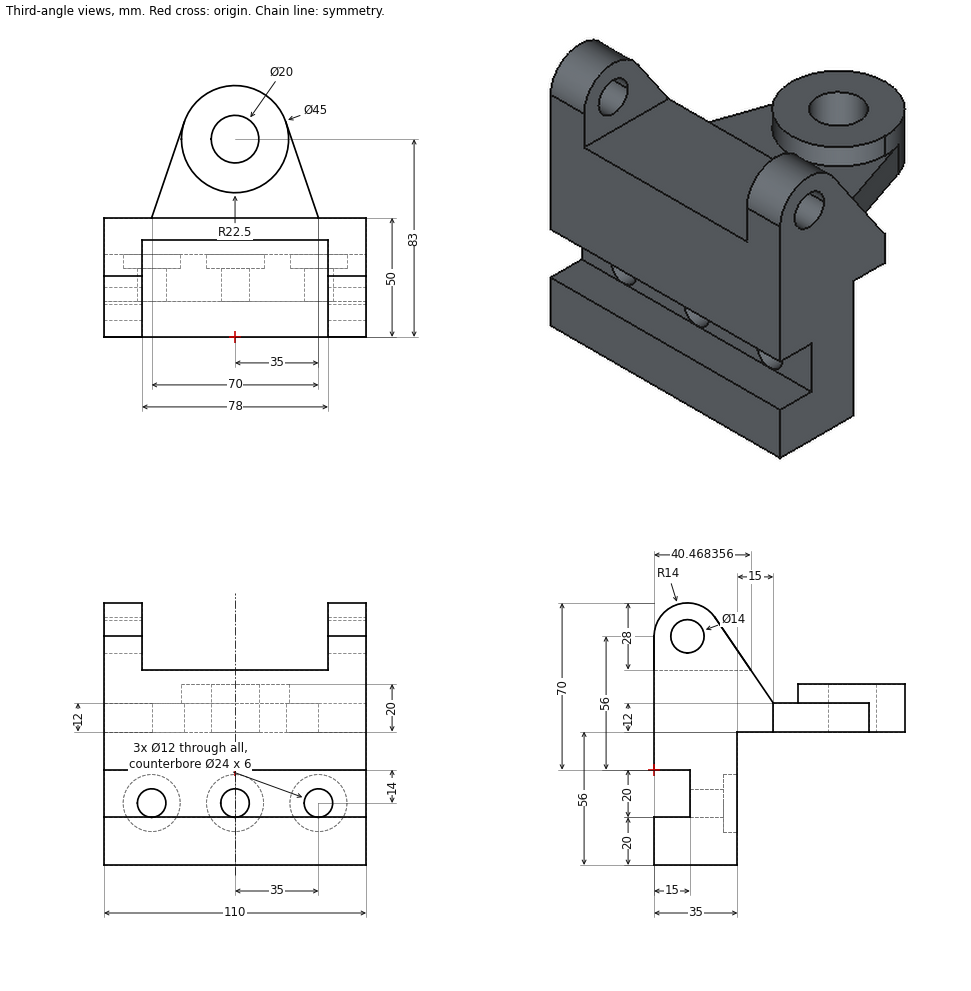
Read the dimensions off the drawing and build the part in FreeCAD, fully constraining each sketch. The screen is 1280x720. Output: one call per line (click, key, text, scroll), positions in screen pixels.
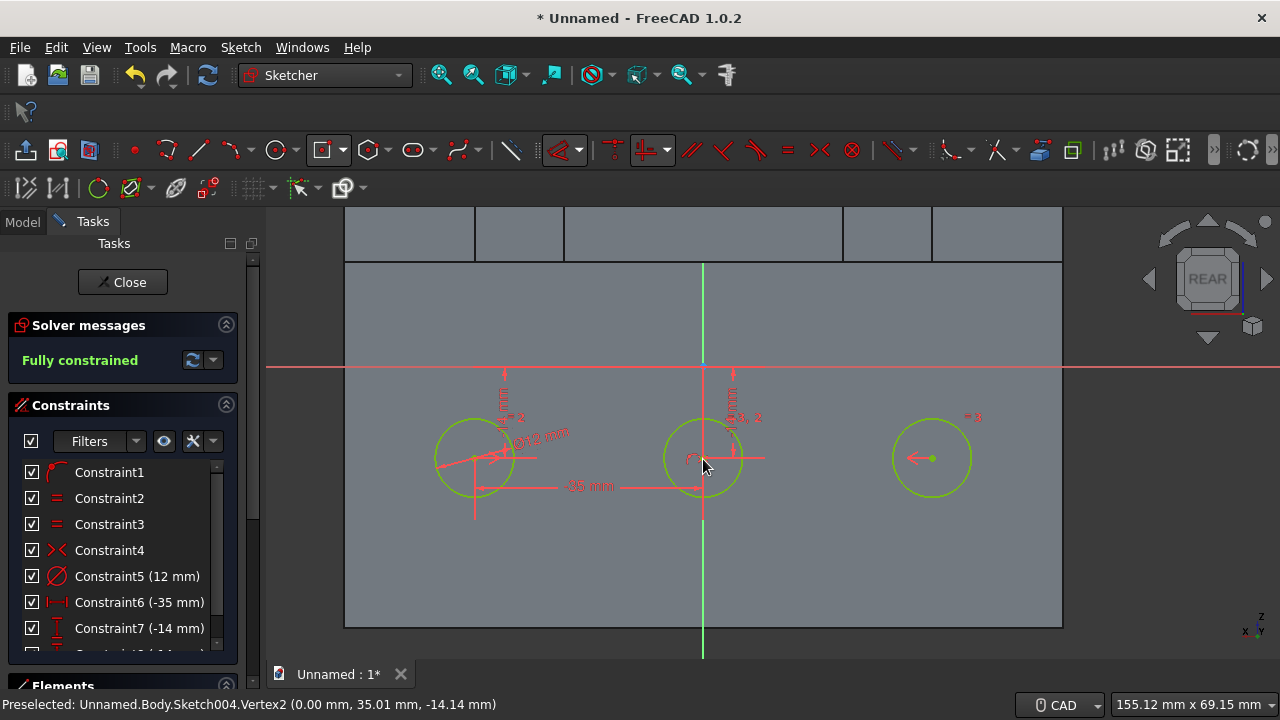
click(123, 282)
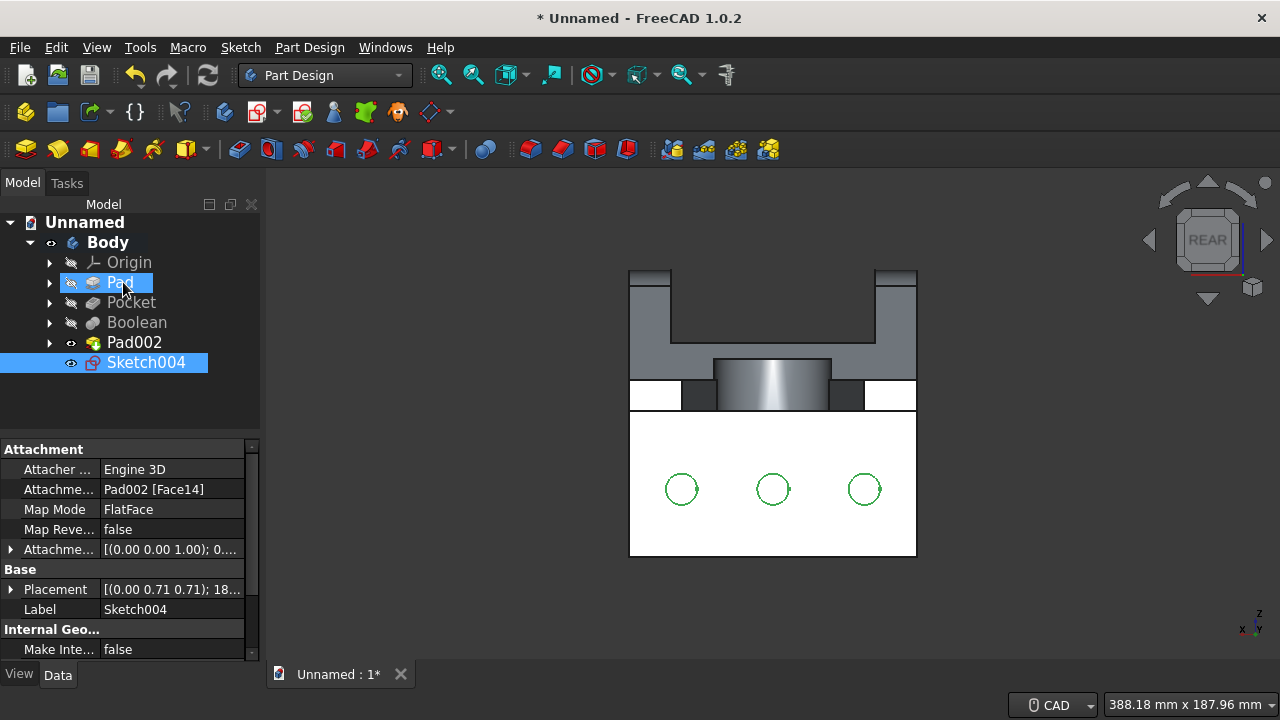
click(272, 150)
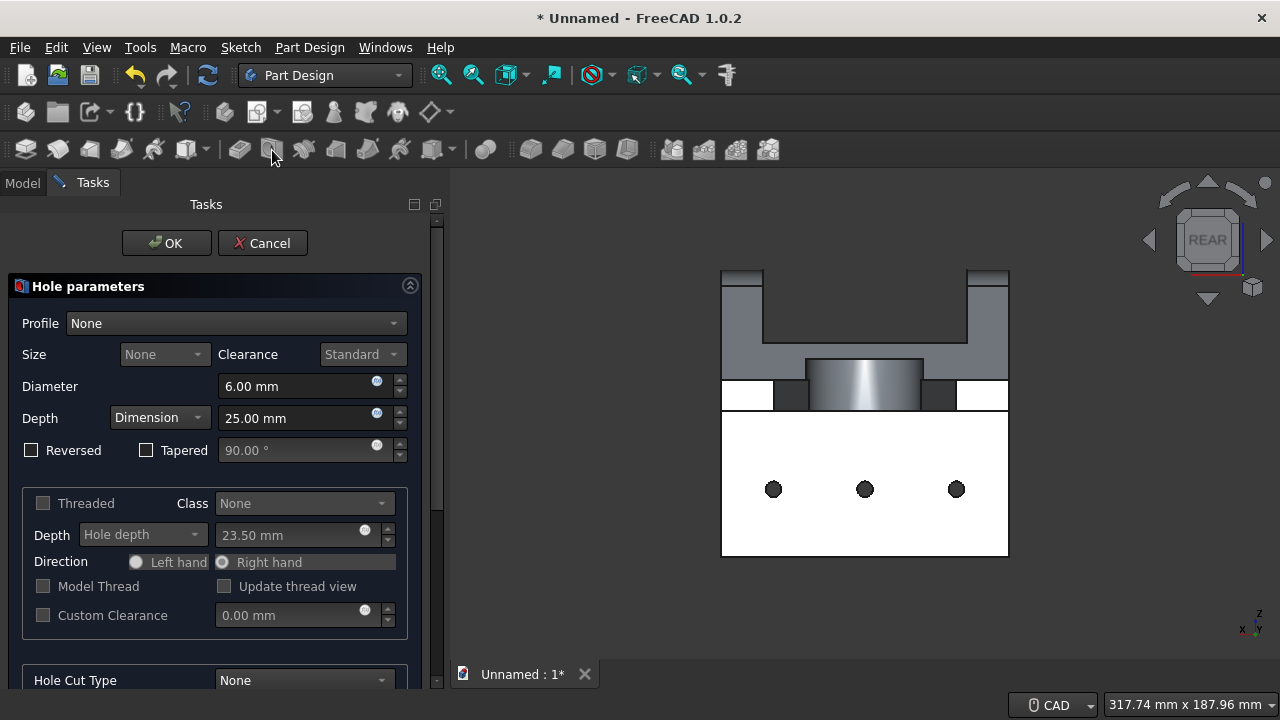
triple_click(305, 386)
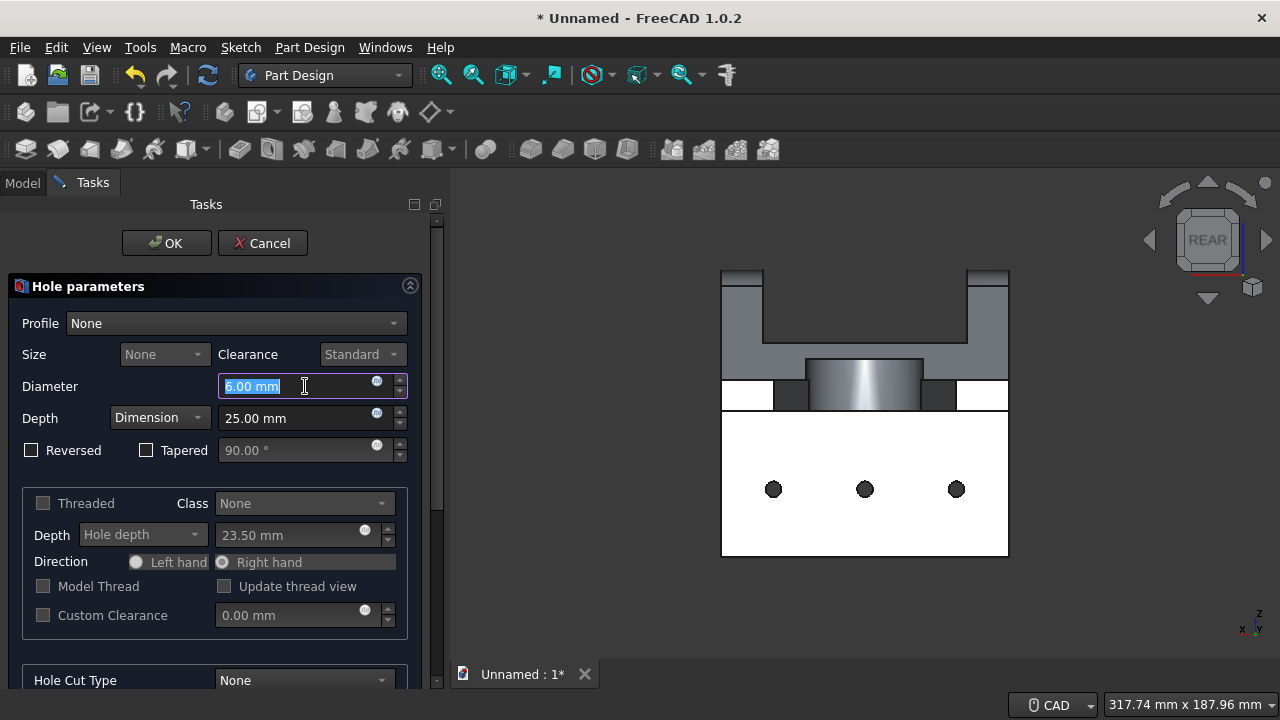
text(12)
key(Tab)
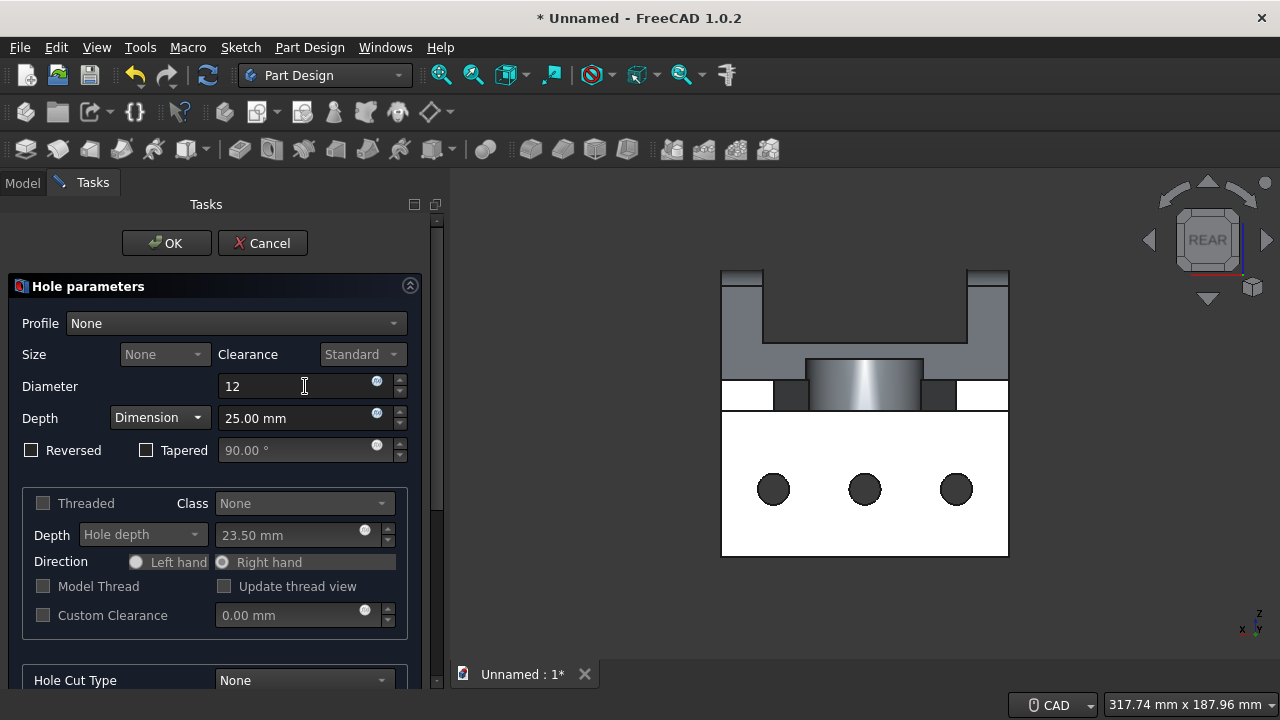
click(161, 418)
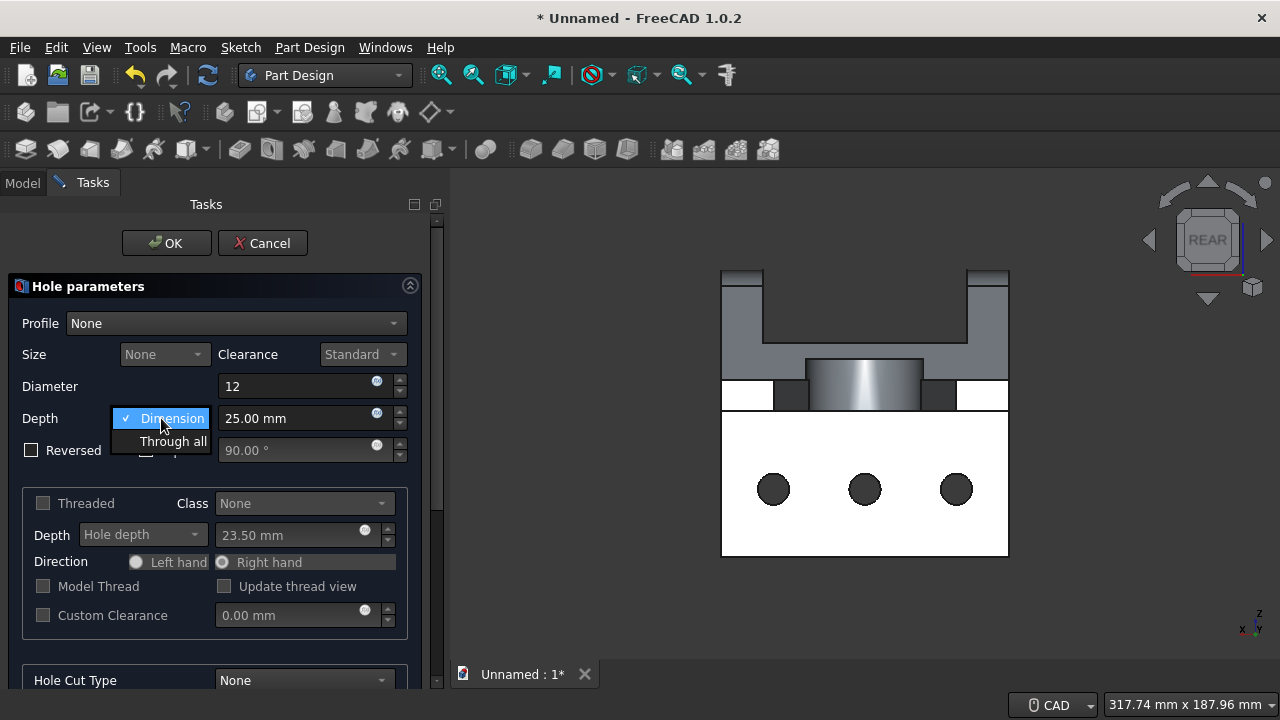
click(160, 442)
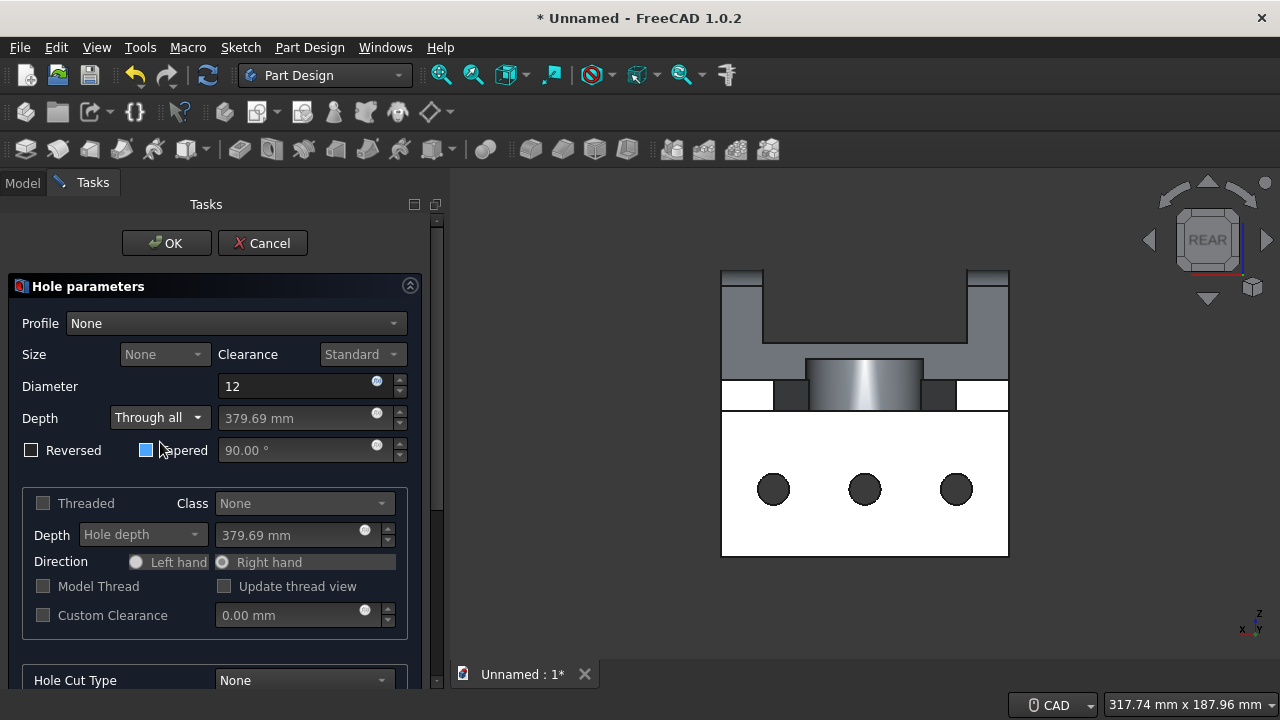
scroll(437, 451, down, 2)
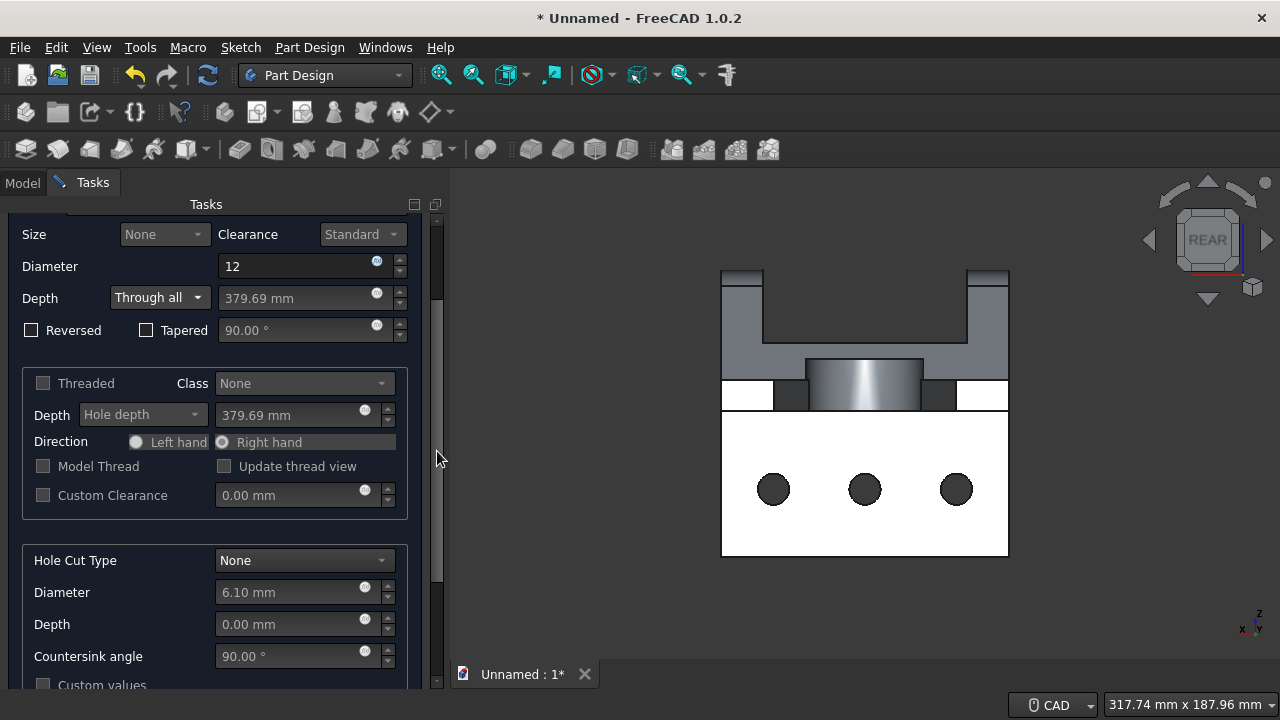
click(306, 560)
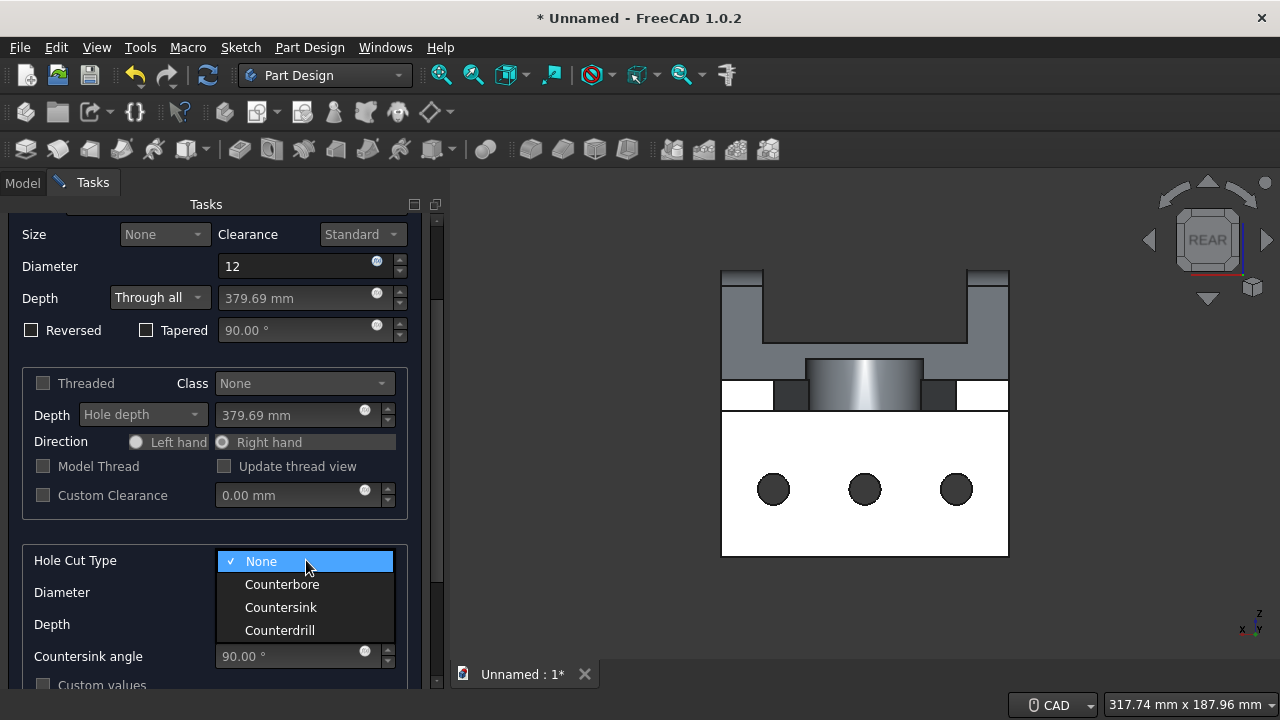
click(304, 584)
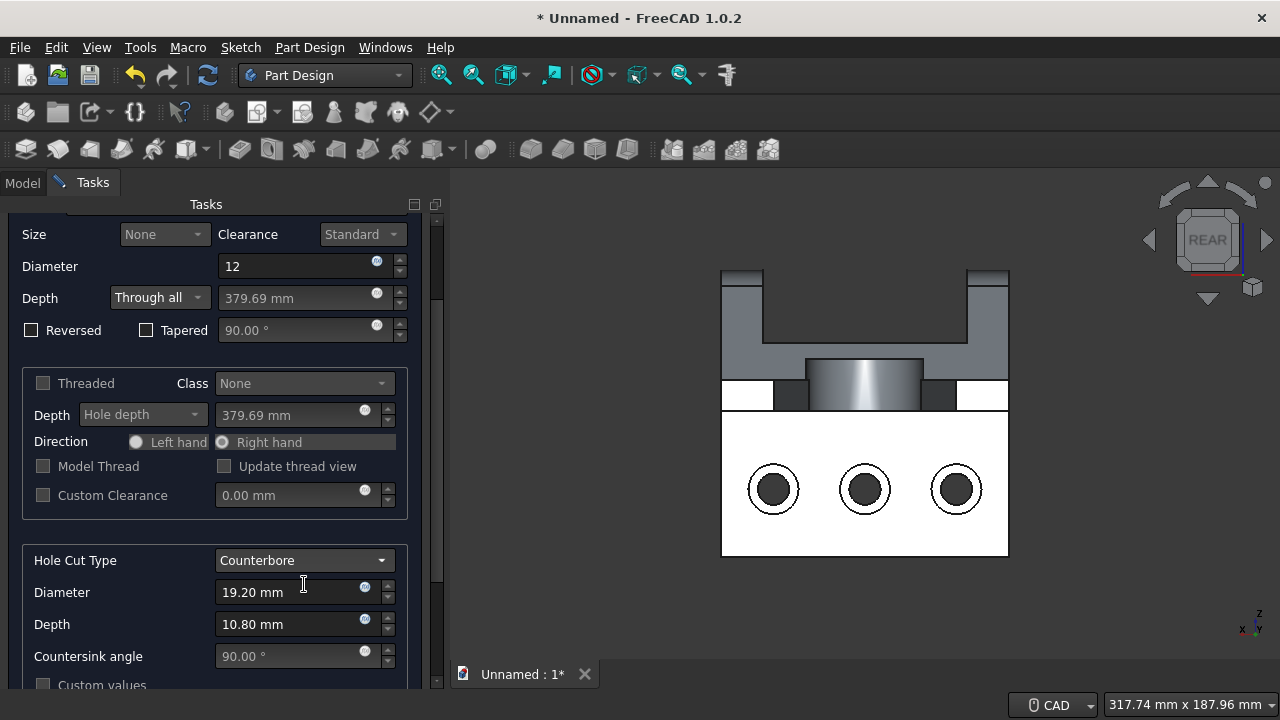
triple_click(298, 592)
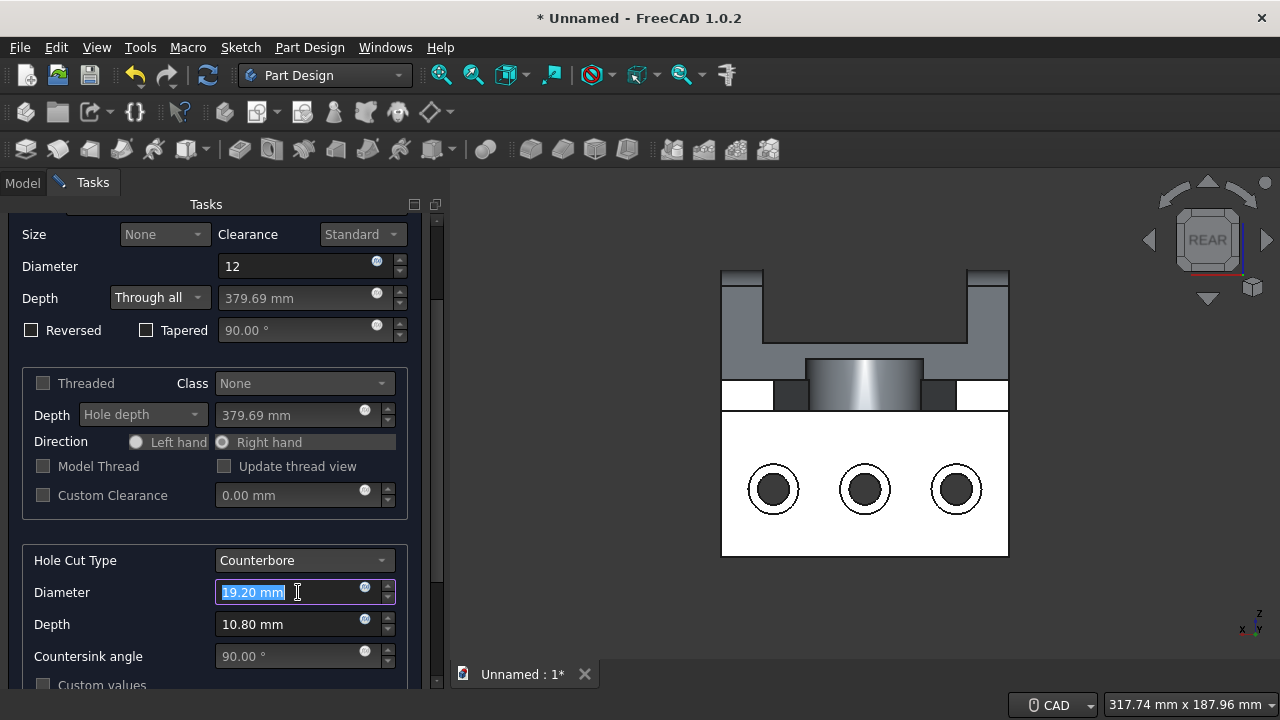
text(24)
key(Tab)